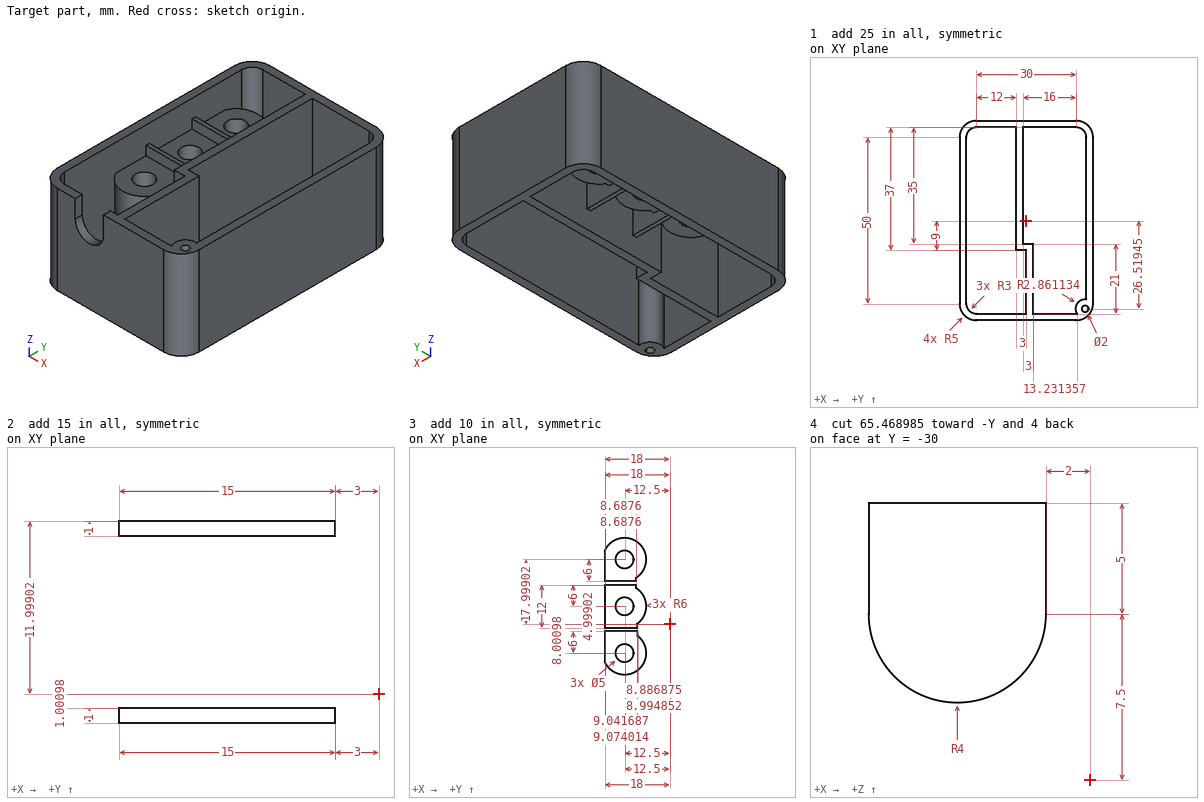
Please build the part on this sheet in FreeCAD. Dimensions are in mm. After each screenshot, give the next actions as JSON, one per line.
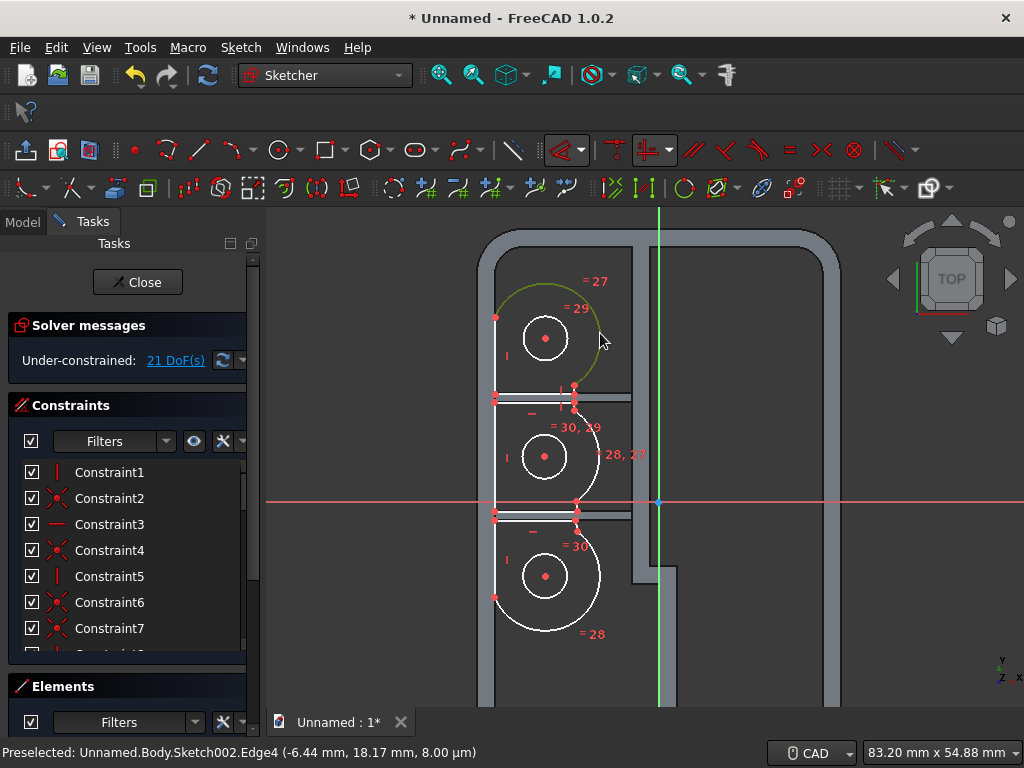
{"action": "left_click", "coordinate": [584, 150]}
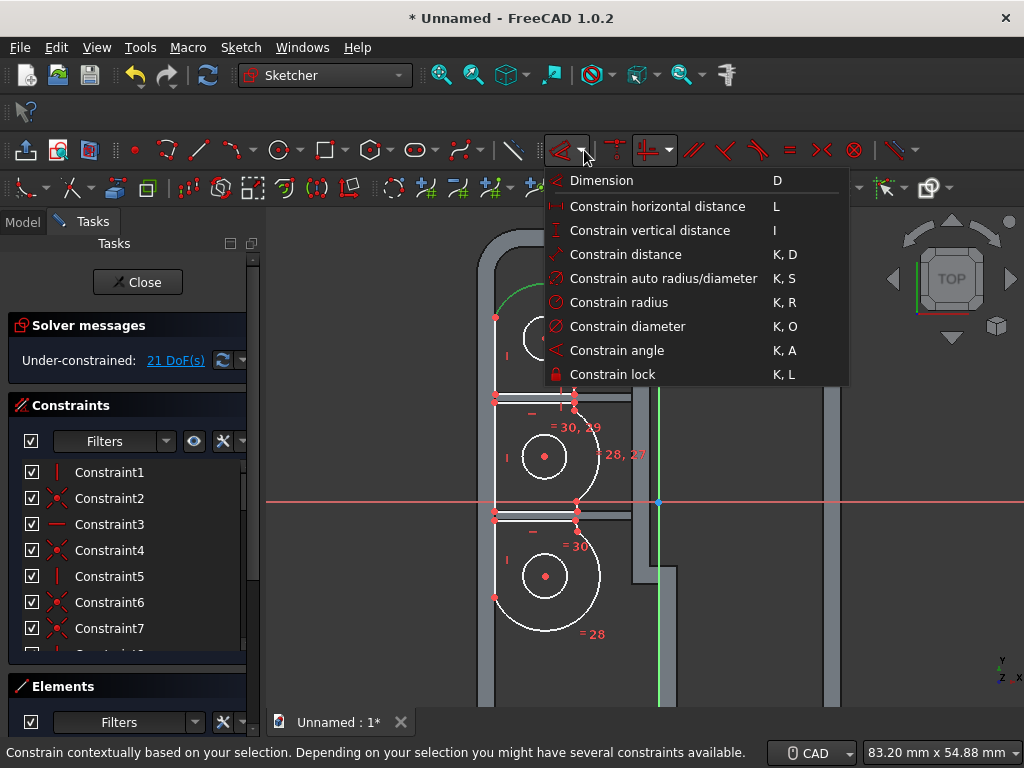
{"action": "left_click", "coordinate": [697, 302]}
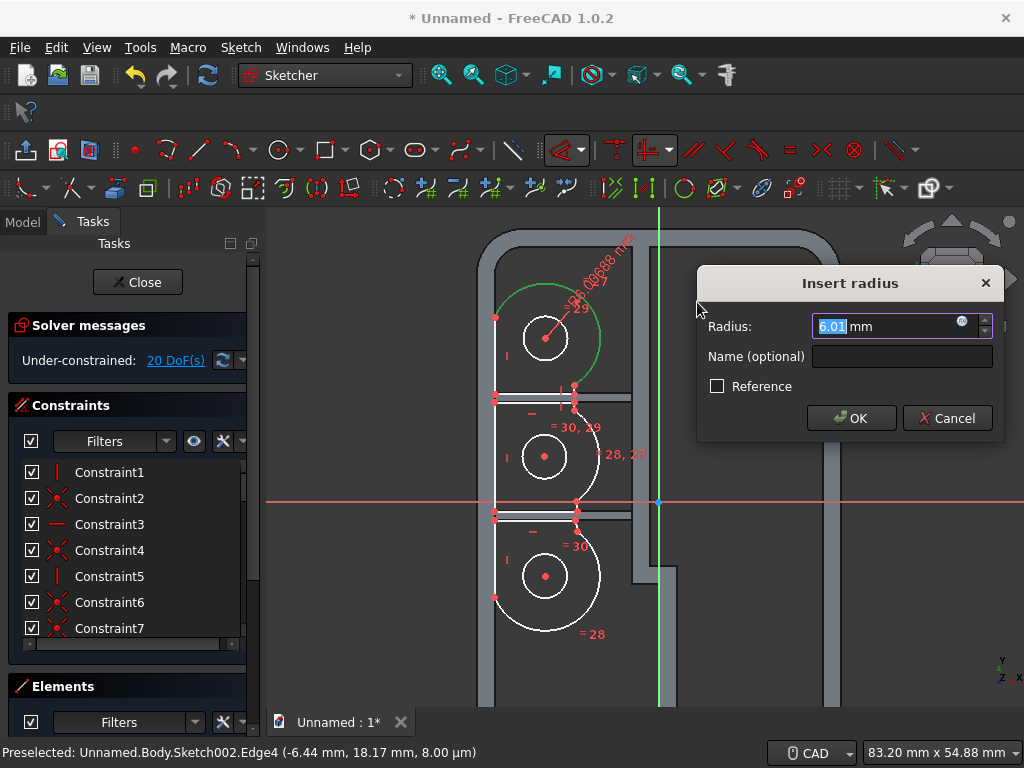
{"action": "type", "text": "6"}
{"action": "key", "text": "Return"}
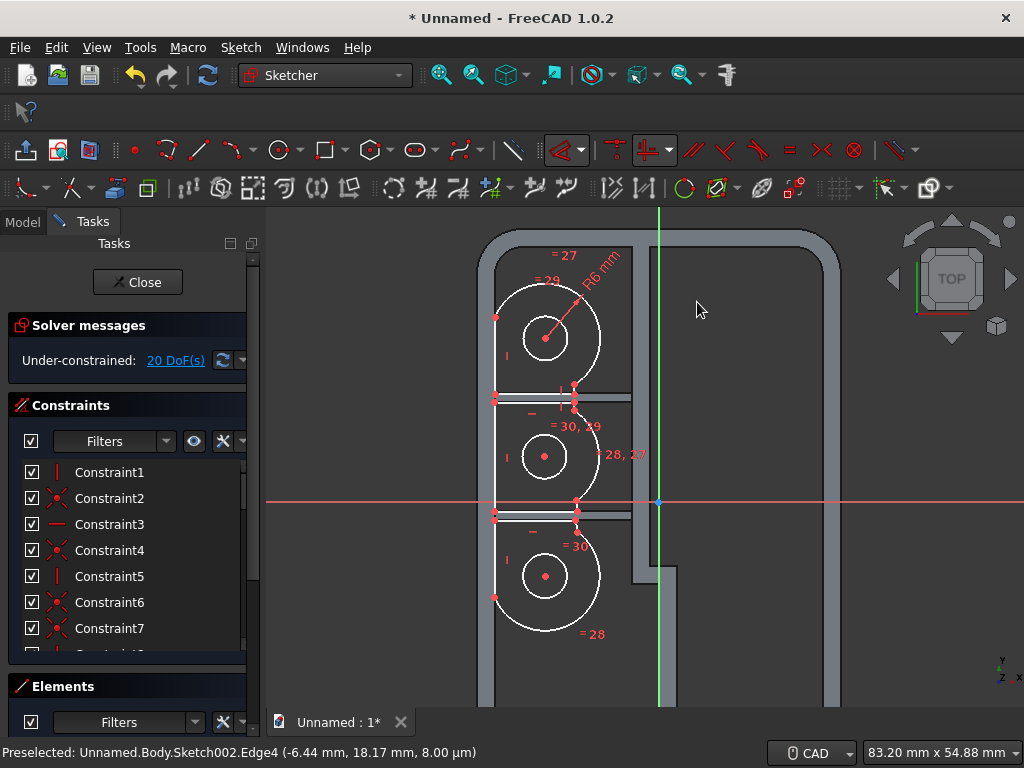
{"action": "left_click", "coordinate": [561, 323]}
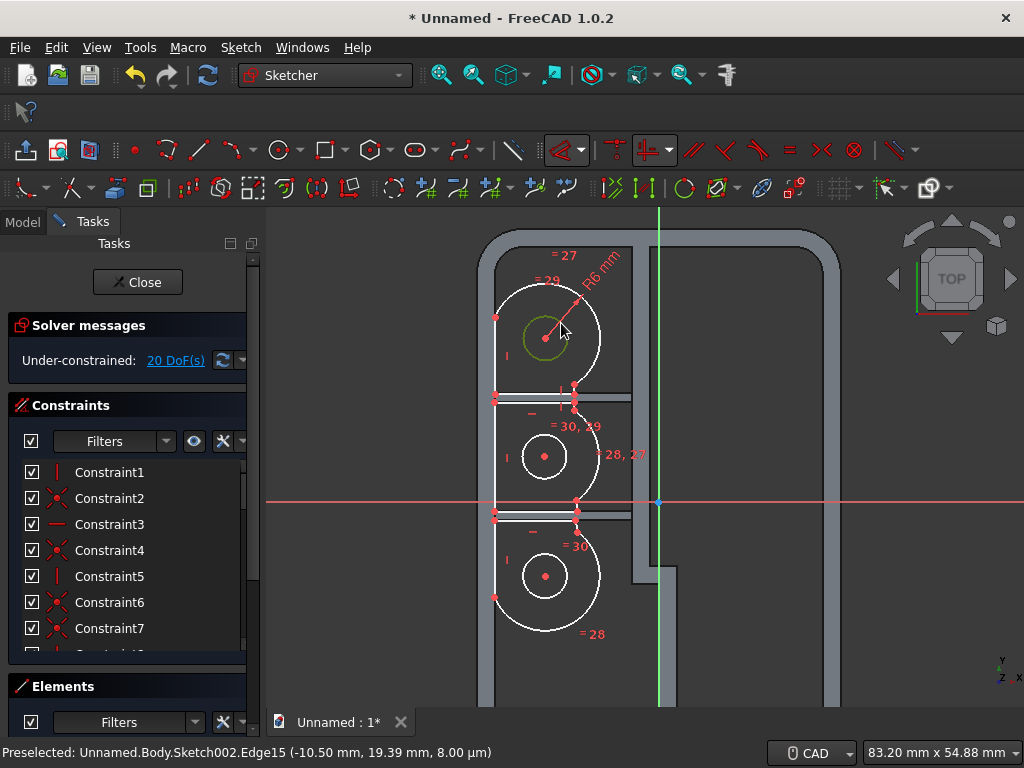
{"action": "left_click", "coordinate": [584, 150]}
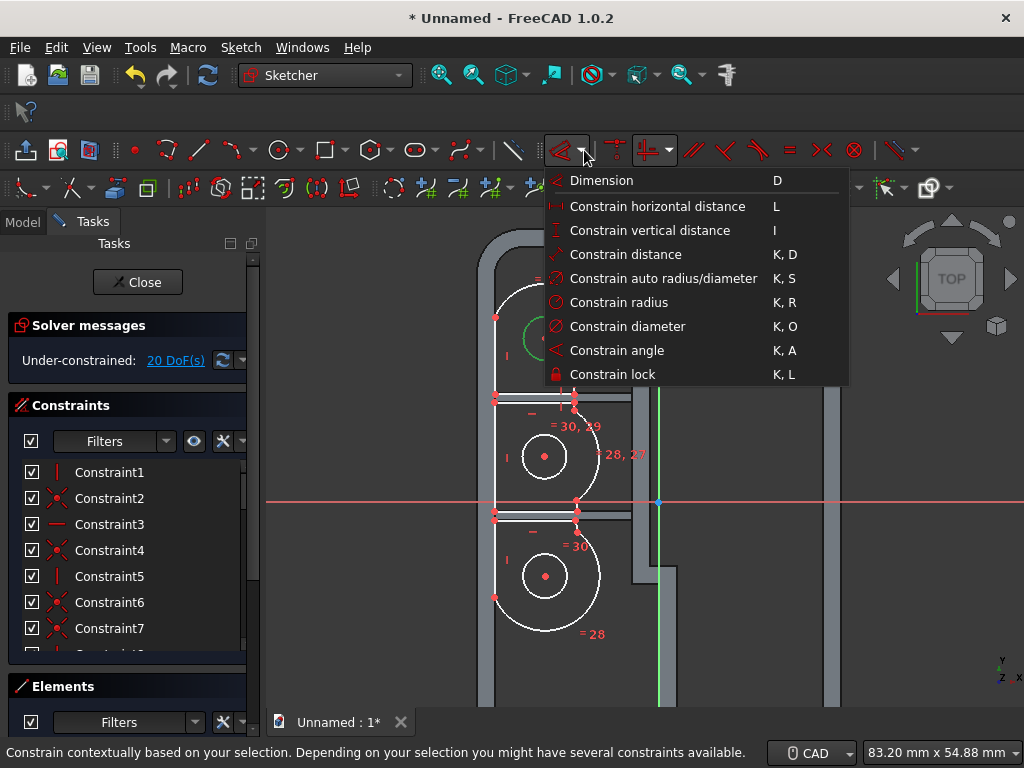
{"action": "left_click", "coordinate": [697, 326]}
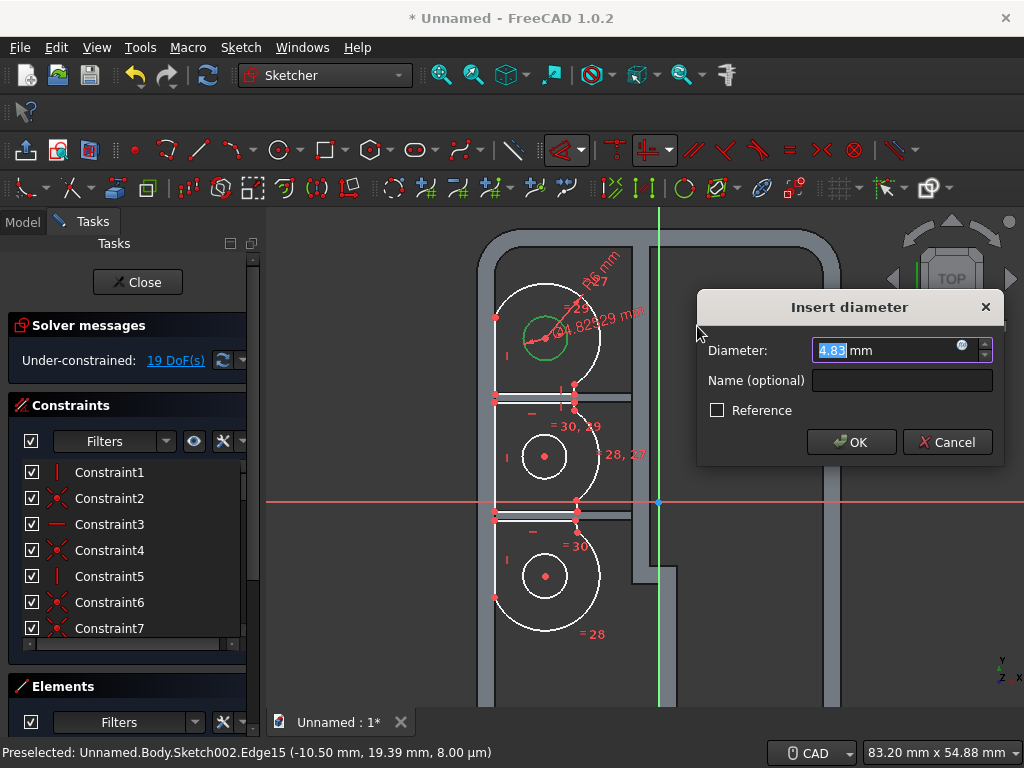
{"action": "type", "text": "5"}
{"action": "key", "text": "Return"}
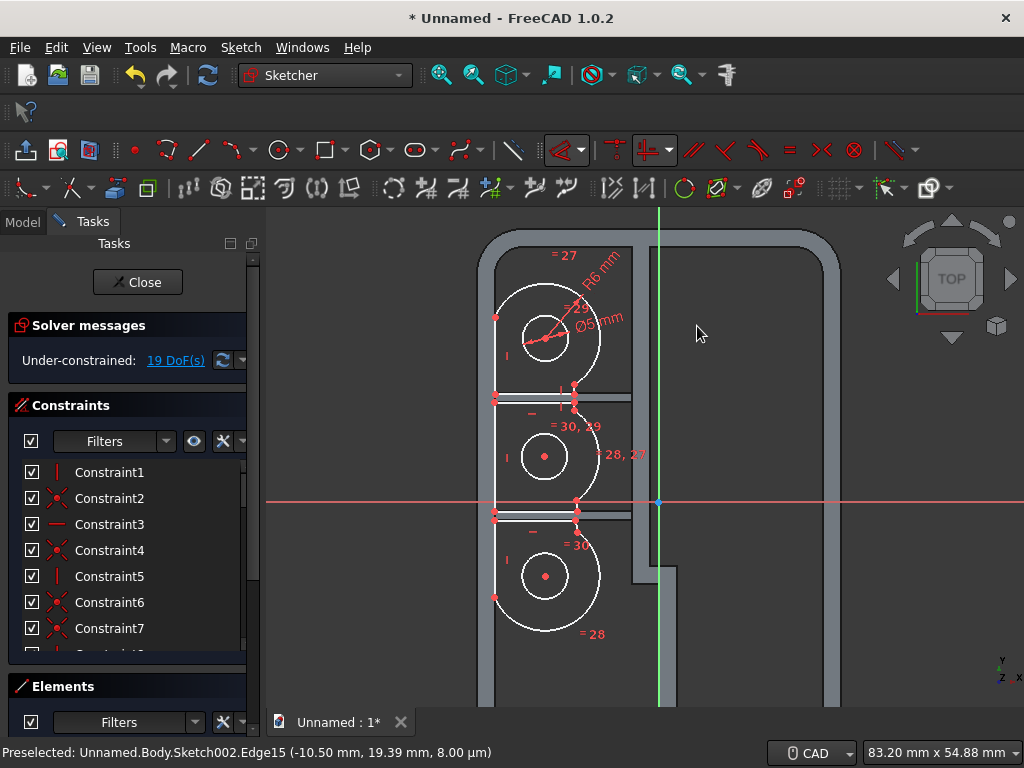
{"action": "left_click", "coordinate": [495, 435]}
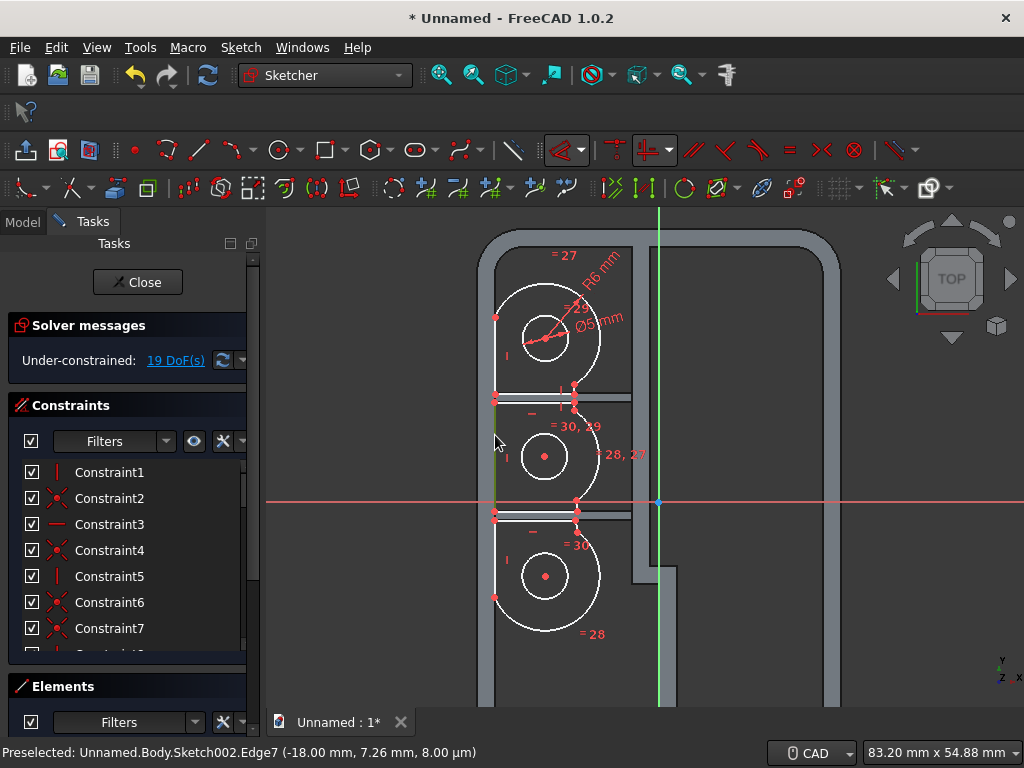
{"action": "key", "text": "i"}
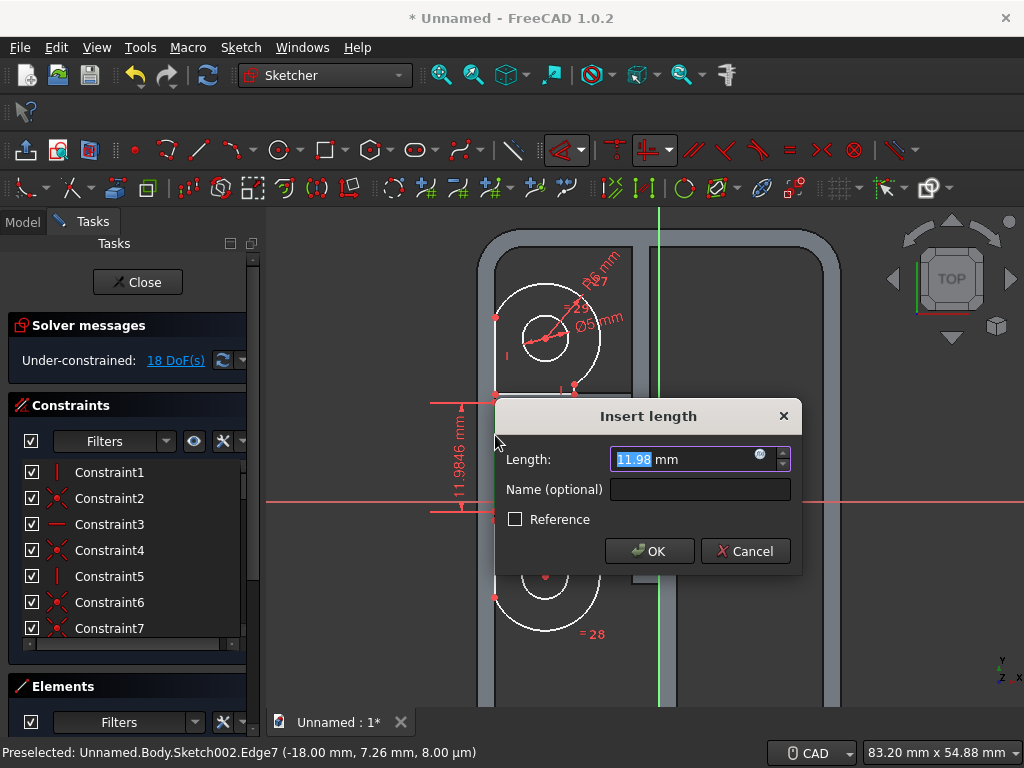
{"action": "type", "text": "12"}
{"action": "key", "text": "Return"}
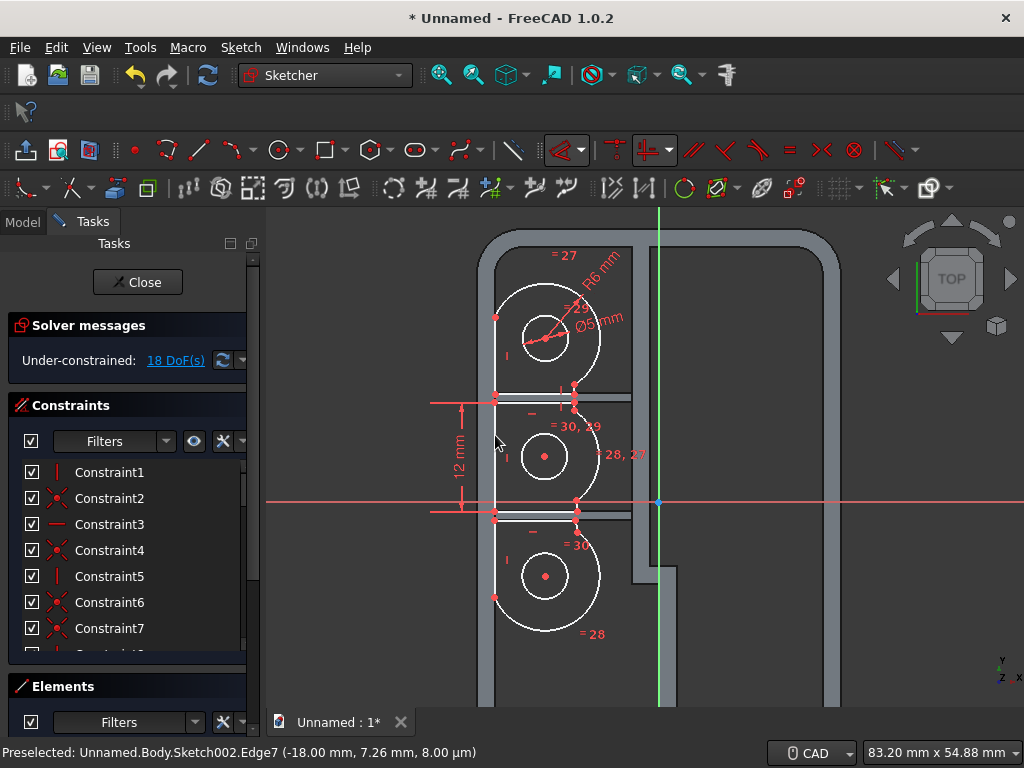
{"action": "scroll", "coordinate": [574, 394], "scroll_direction": "up", "scroll_amount": 2}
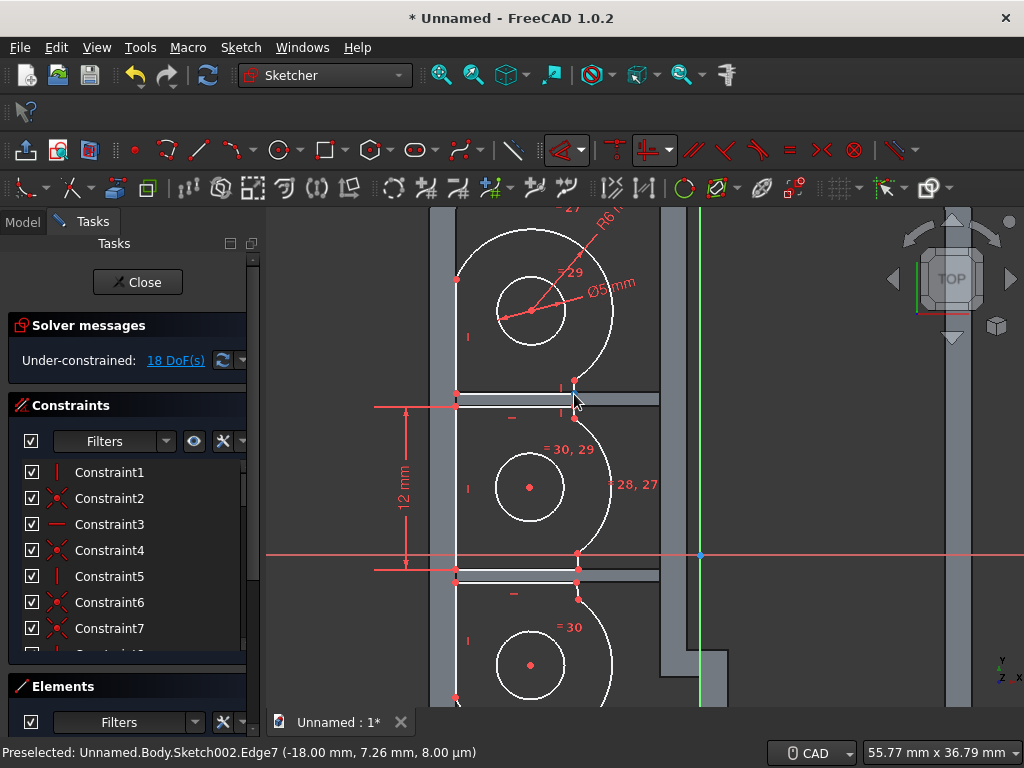
{"action": "left_click", "coordinate": [574, 394]}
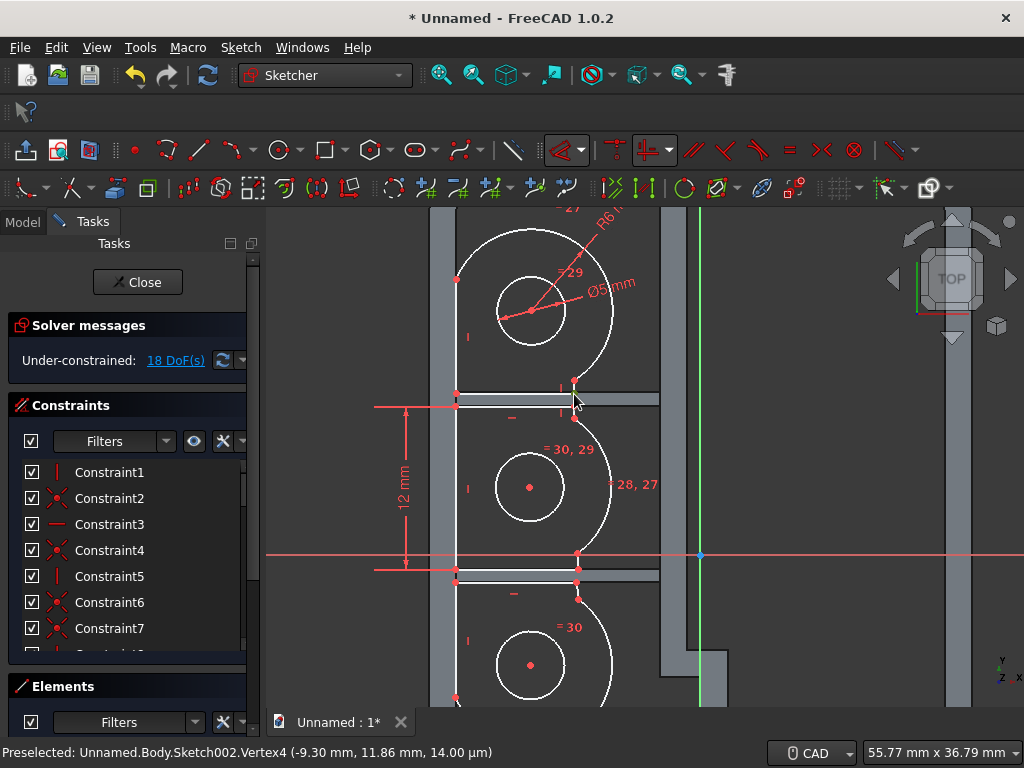
{"action": "left_click", "coordinate": [531, 311]}